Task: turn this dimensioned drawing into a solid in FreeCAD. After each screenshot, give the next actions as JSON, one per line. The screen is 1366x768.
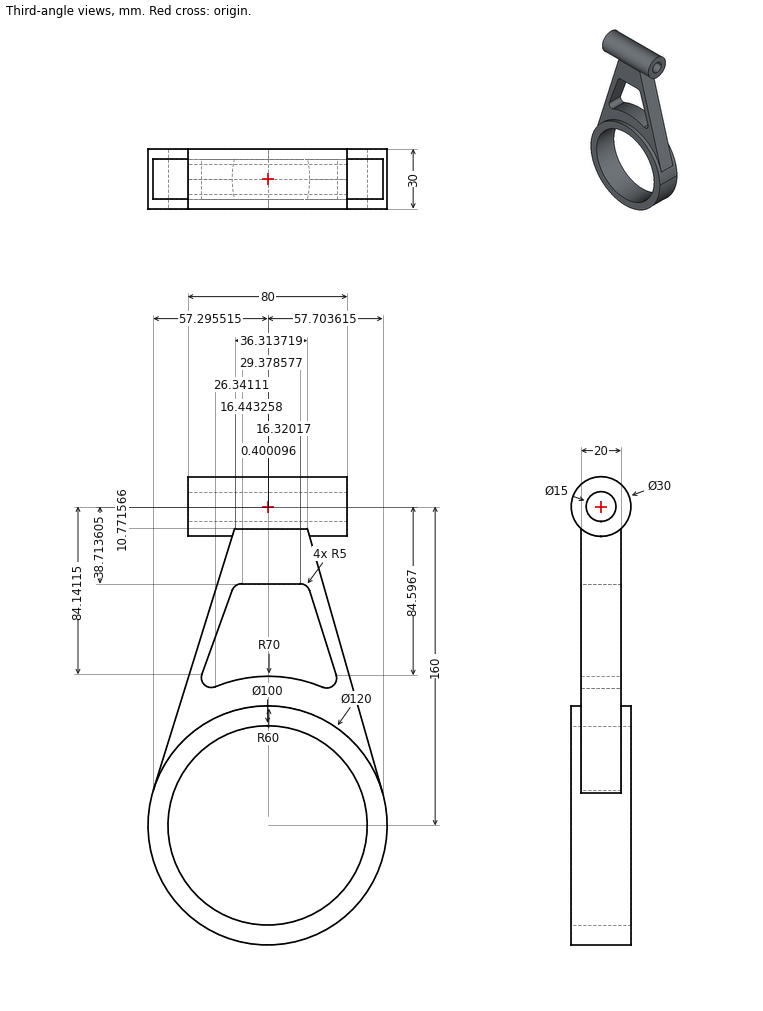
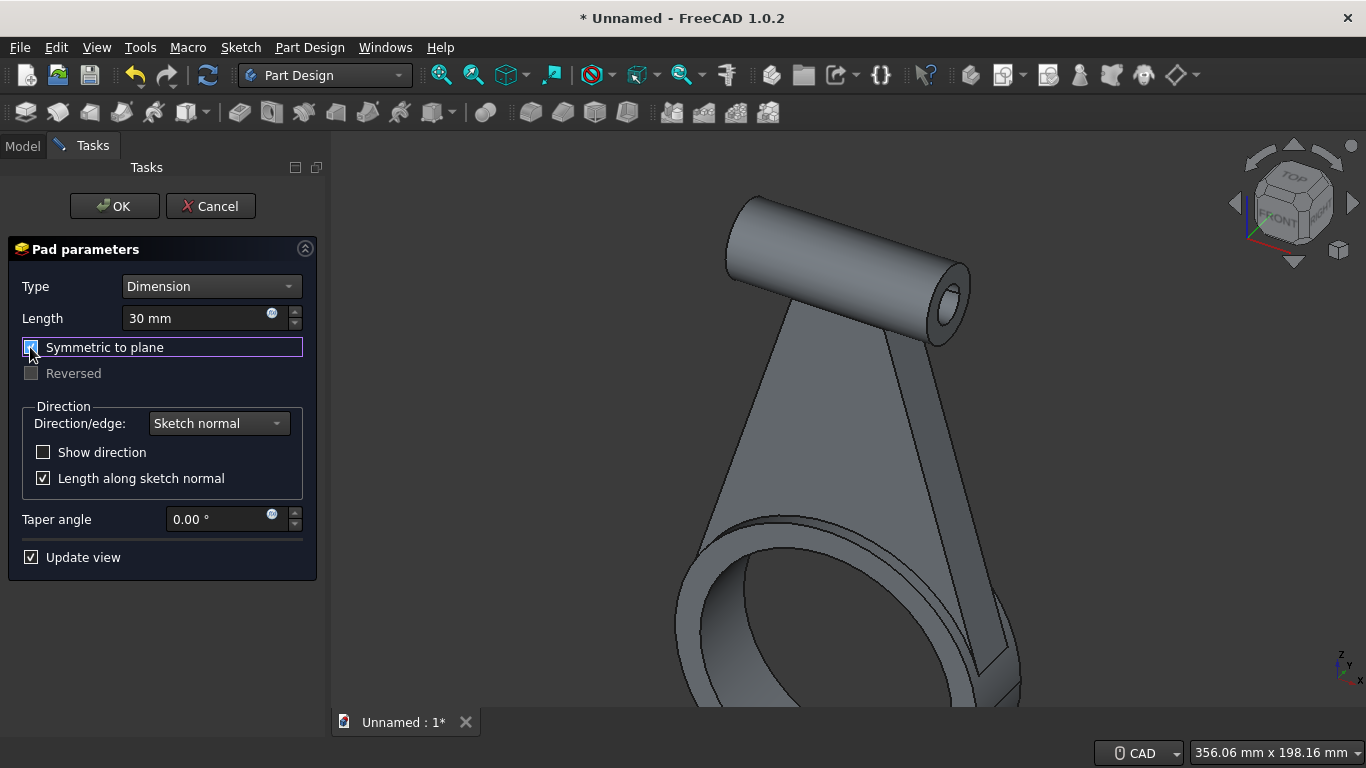
{"action": "left_click", "coordinate": [115, 206]}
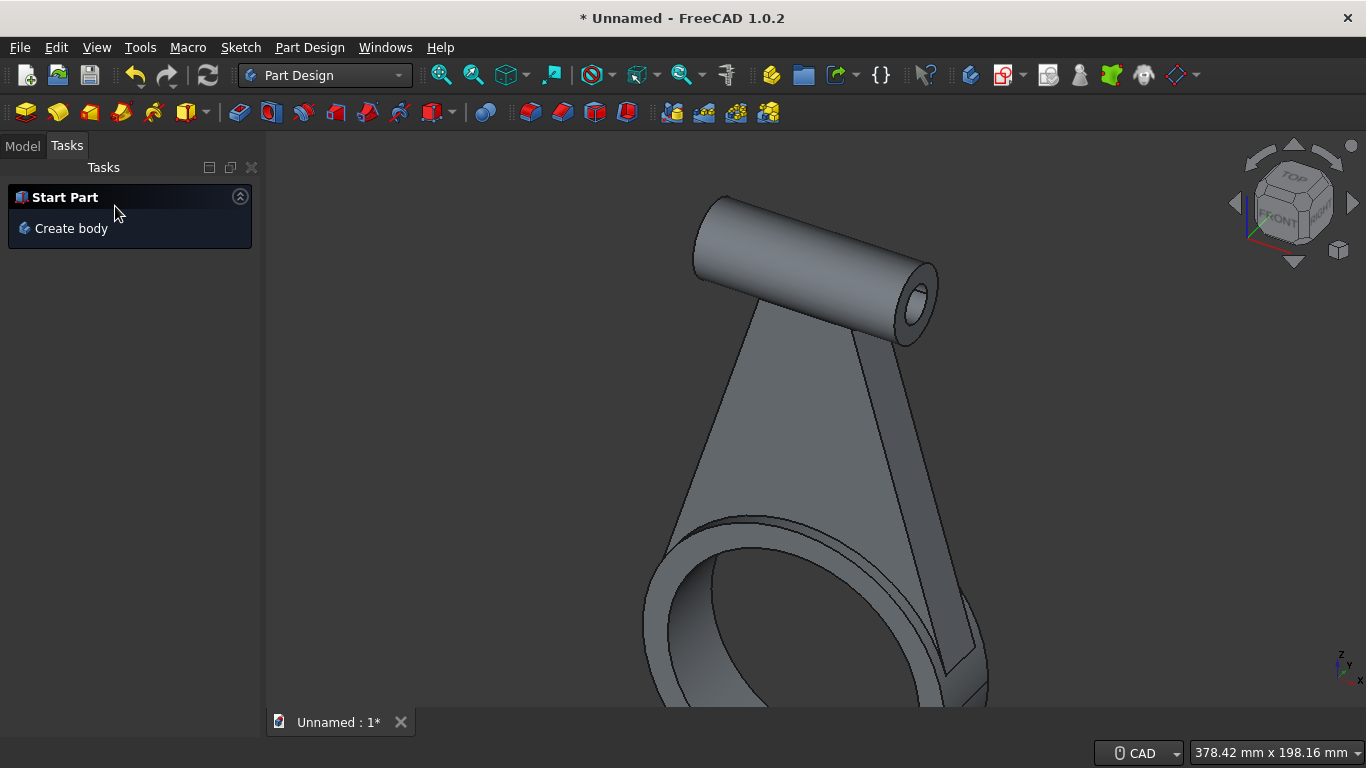
{"action": "left_click", "coordinate": [442, 76]}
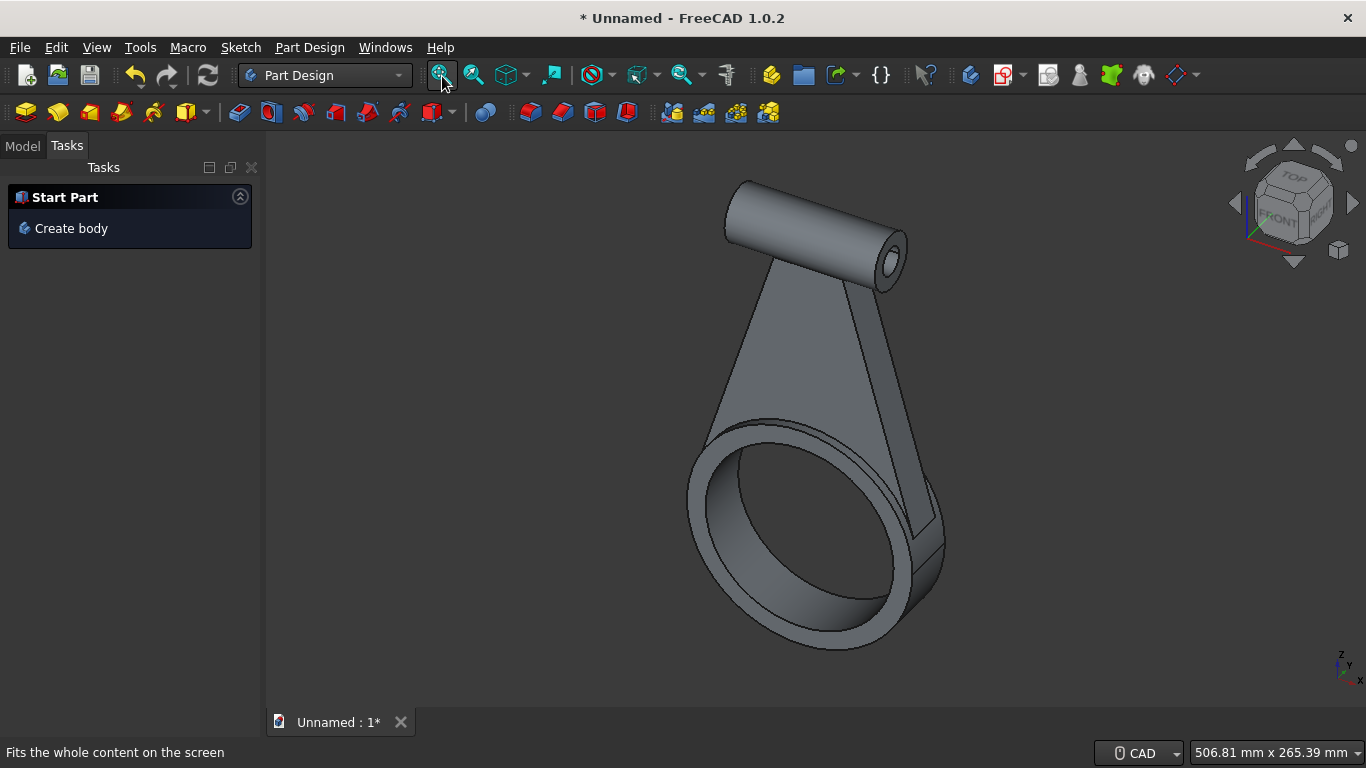
{"action": "key", "text": "4"}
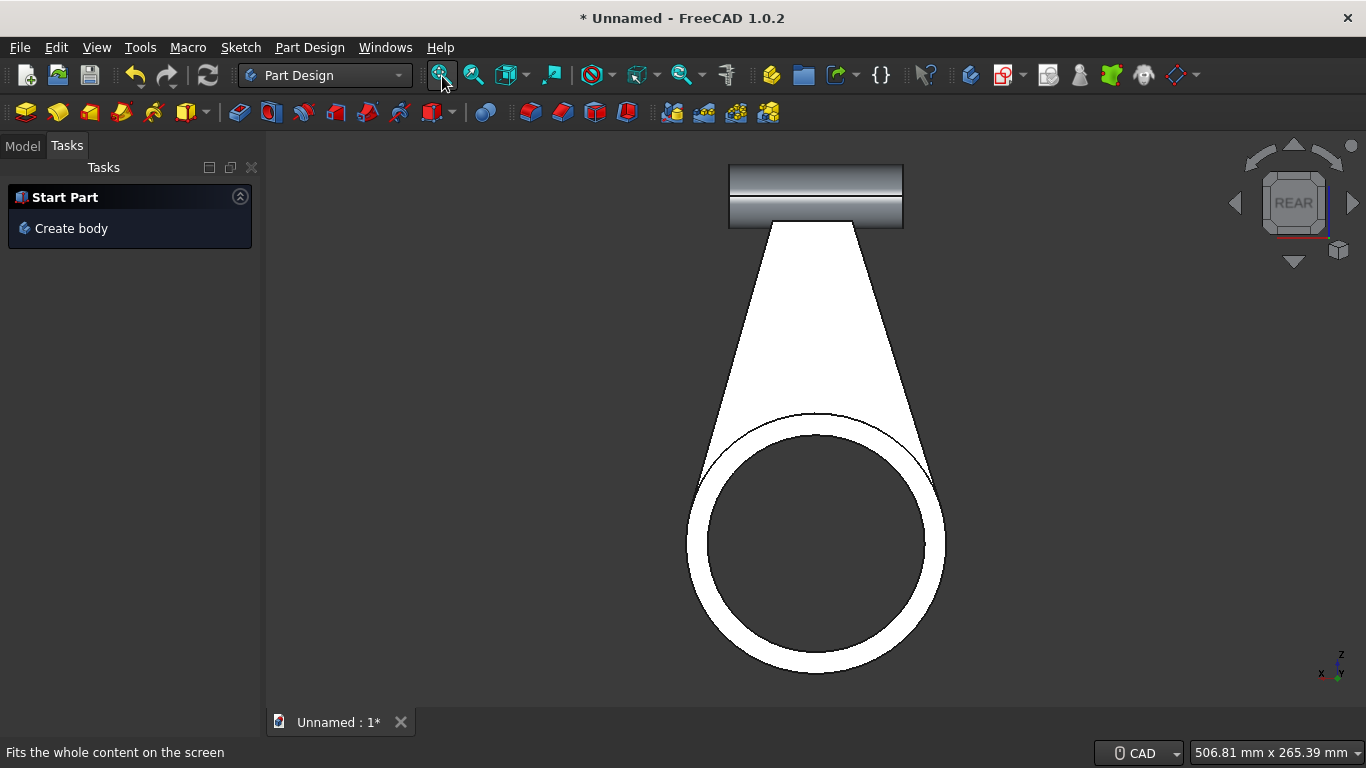
{"action": "left_click", "coordinate": [816, 322]}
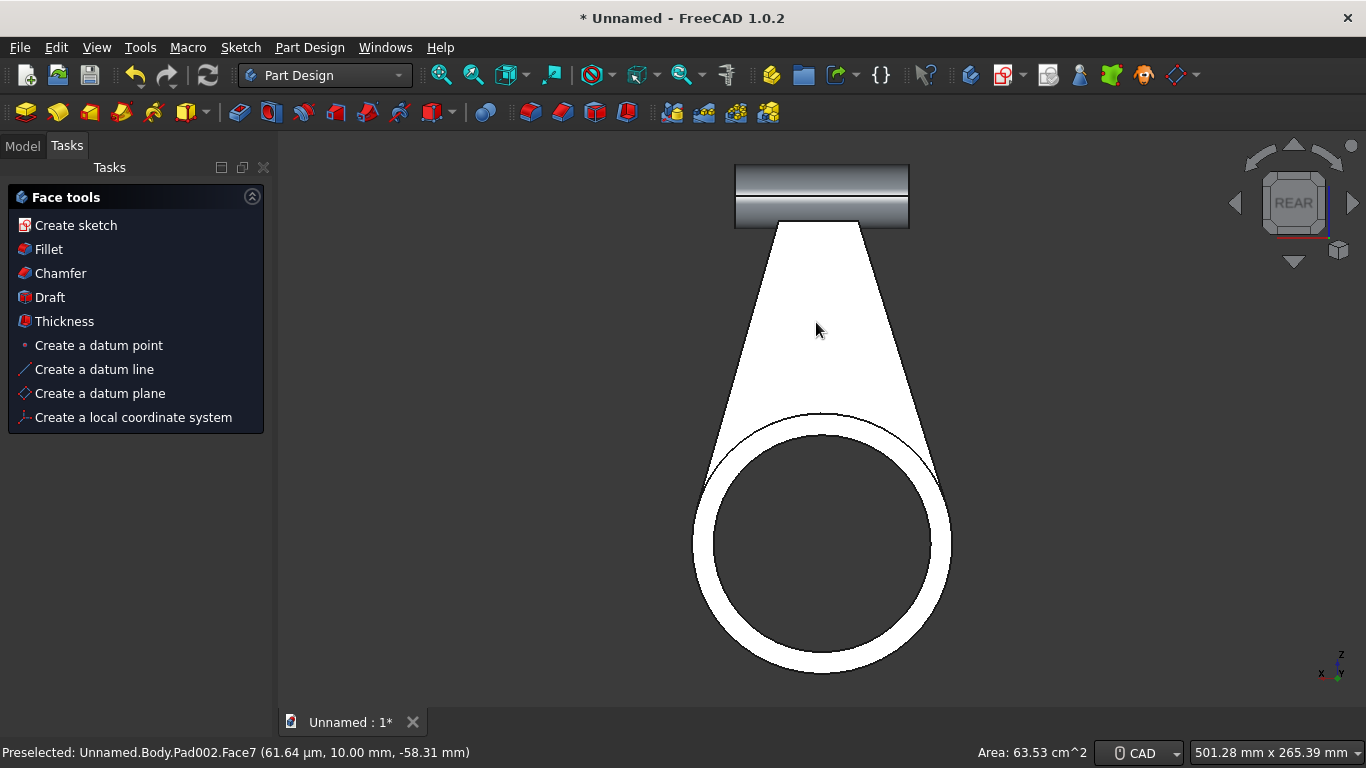
{"action": "left_click", "coordinate": [1004, 76]}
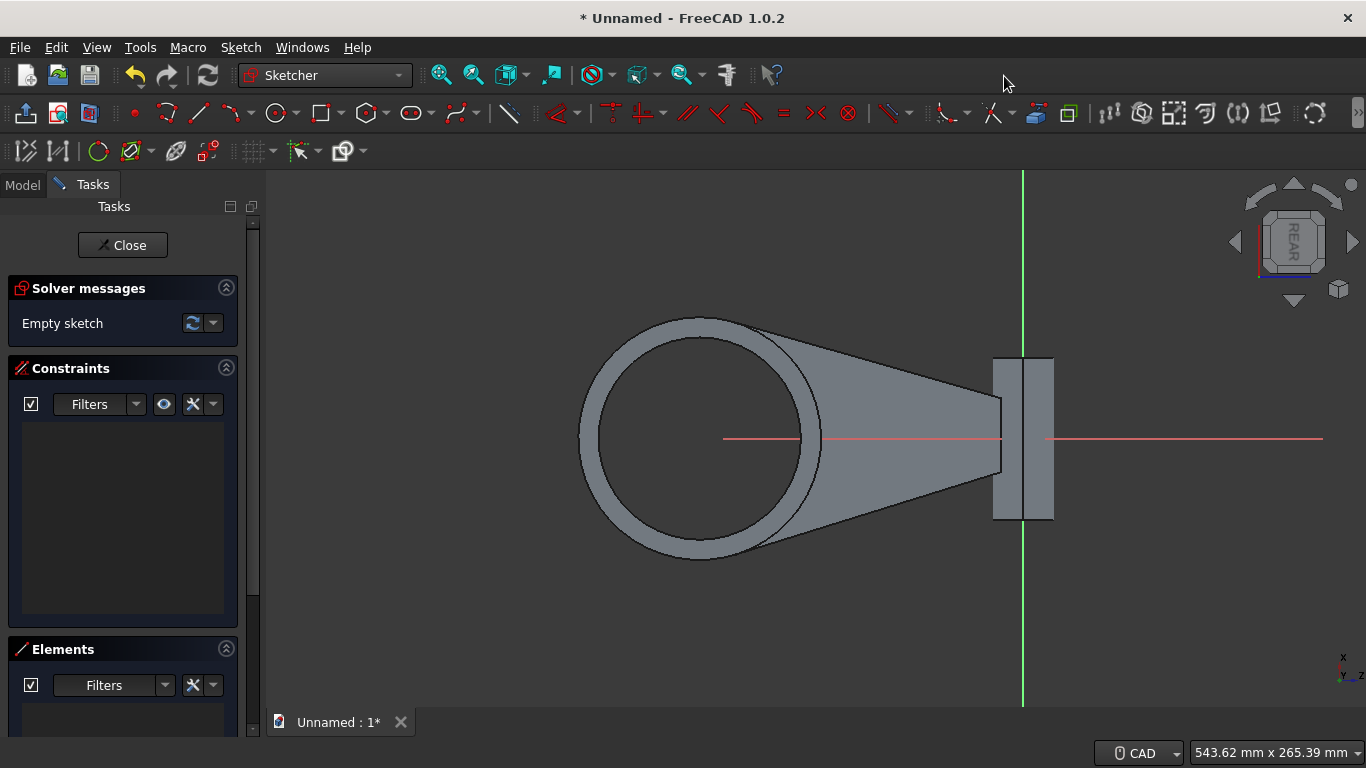
{"action": "left_click", "coordinate": [90, 114]}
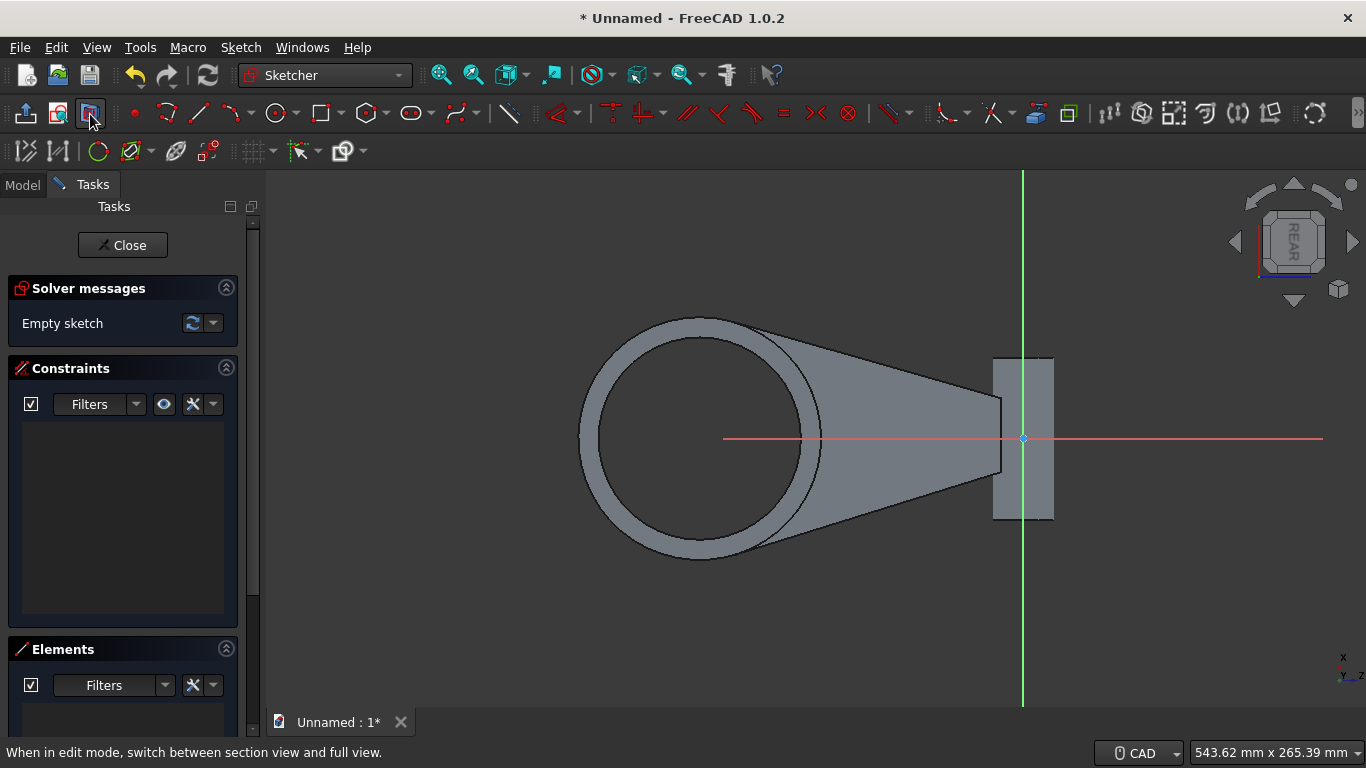
{"action": "scroll", "coordinate": [1039, 436], "scroll_direction": "up", "scroll_amount": 5}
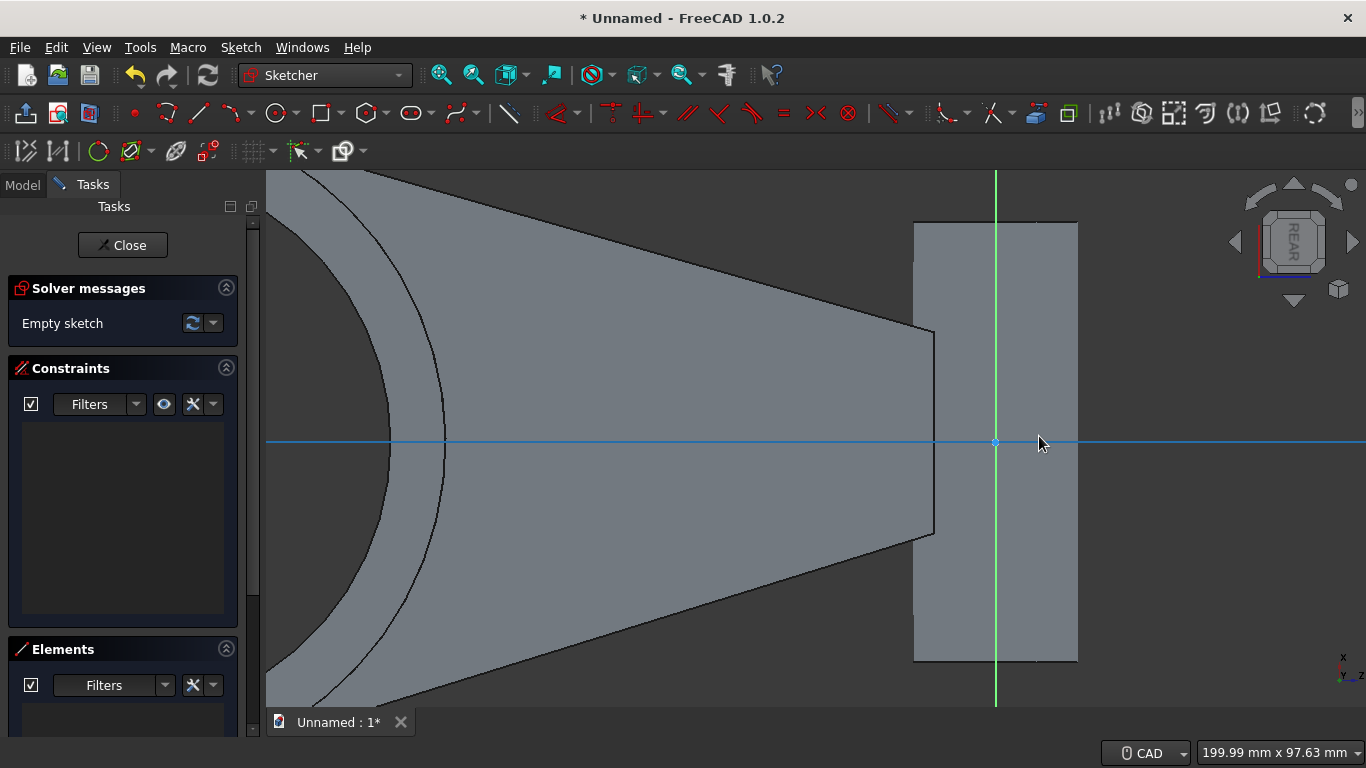
{"action": "left_click", "coordinate": [200, 114]}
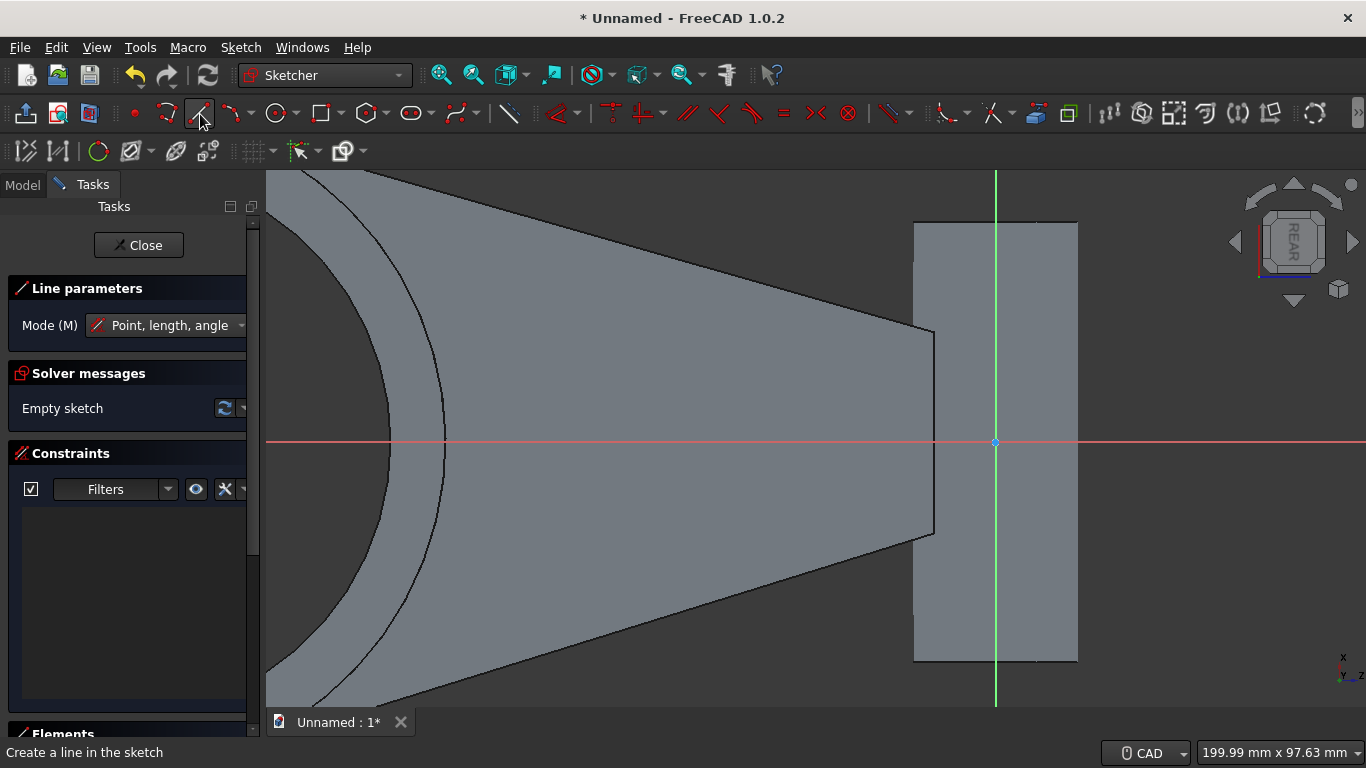
{"action": "left_click", "coordinate": [783, 514]}
{"action": "left_click", "coordinate": [783, 353]}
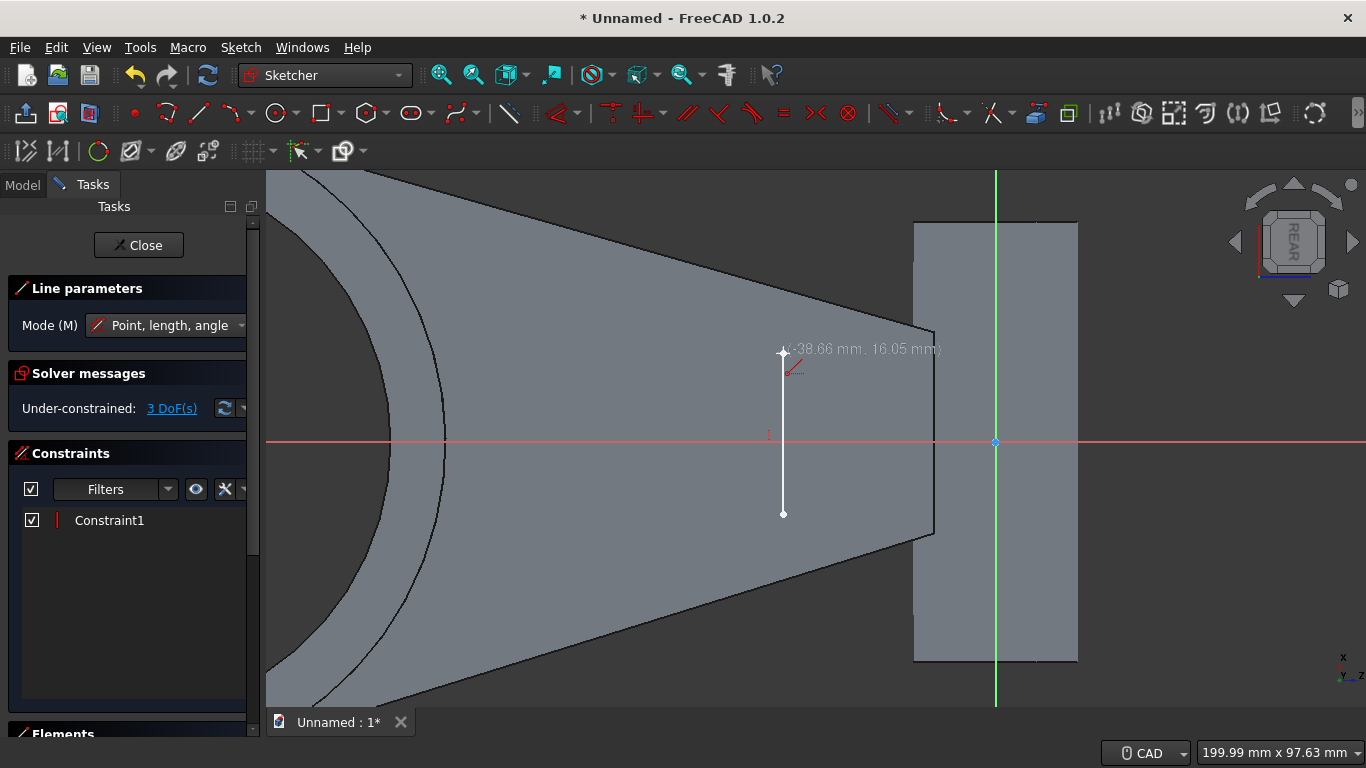
{"action": "left_click", "coordinate": [763, 326]}
{"action": "left_click", "coordinate": [530, 253]}